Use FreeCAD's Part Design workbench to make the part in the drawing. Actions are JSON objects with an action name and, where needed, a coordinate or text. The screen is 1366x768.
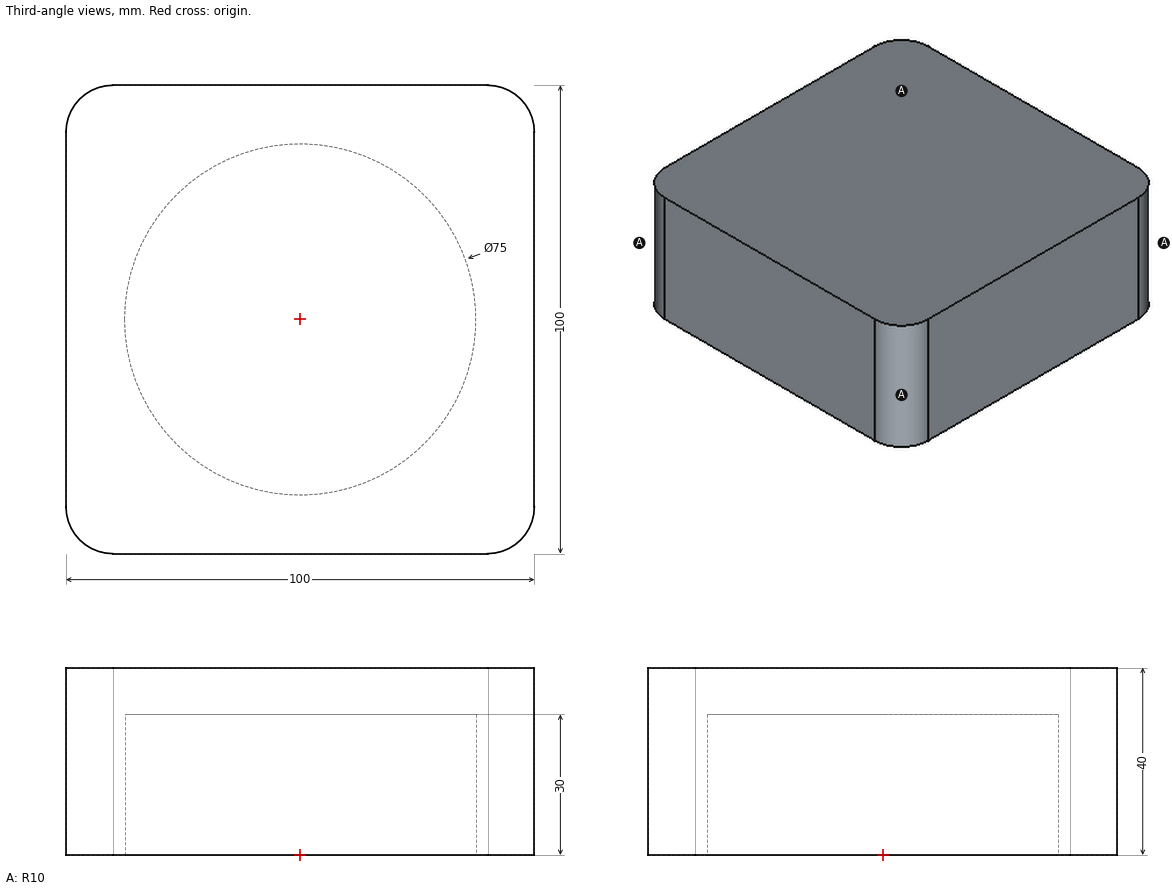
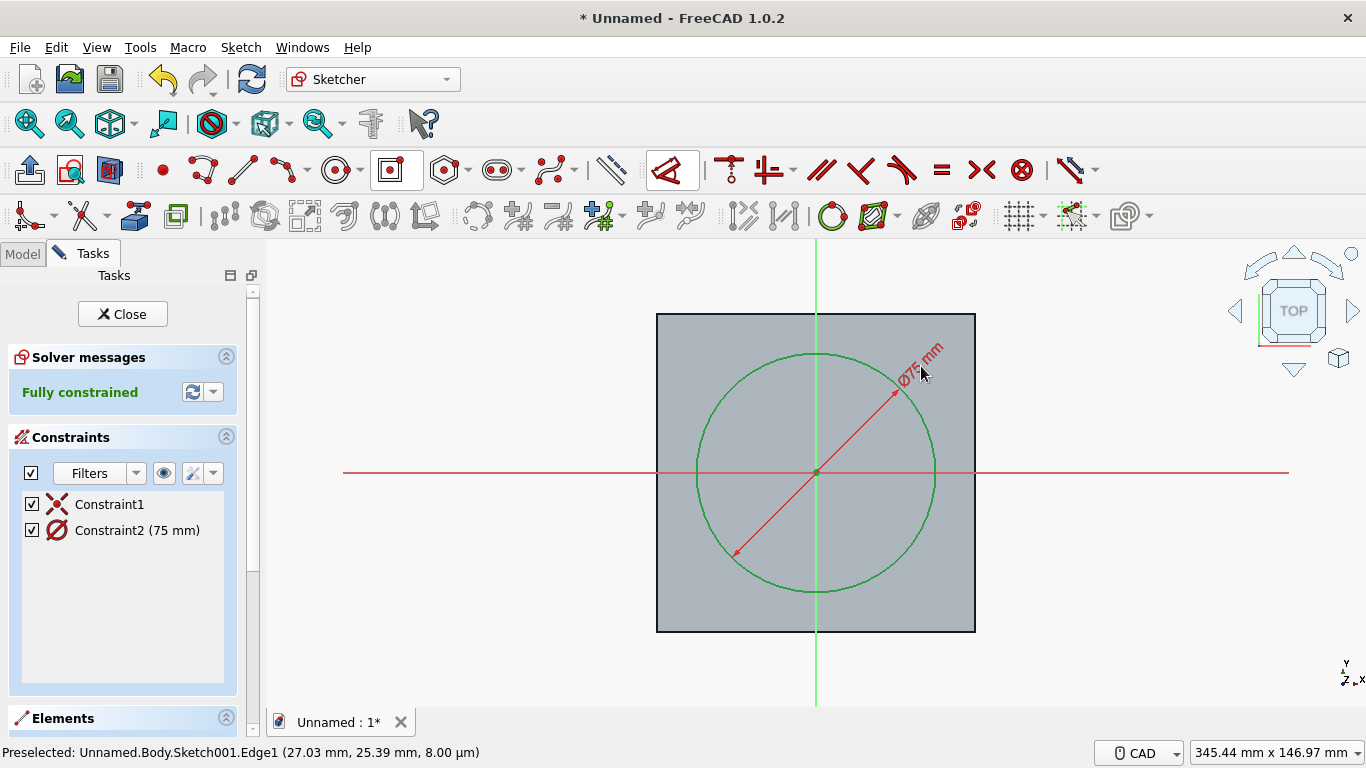
{"action": "left_click", "coordinate": [123, 314]}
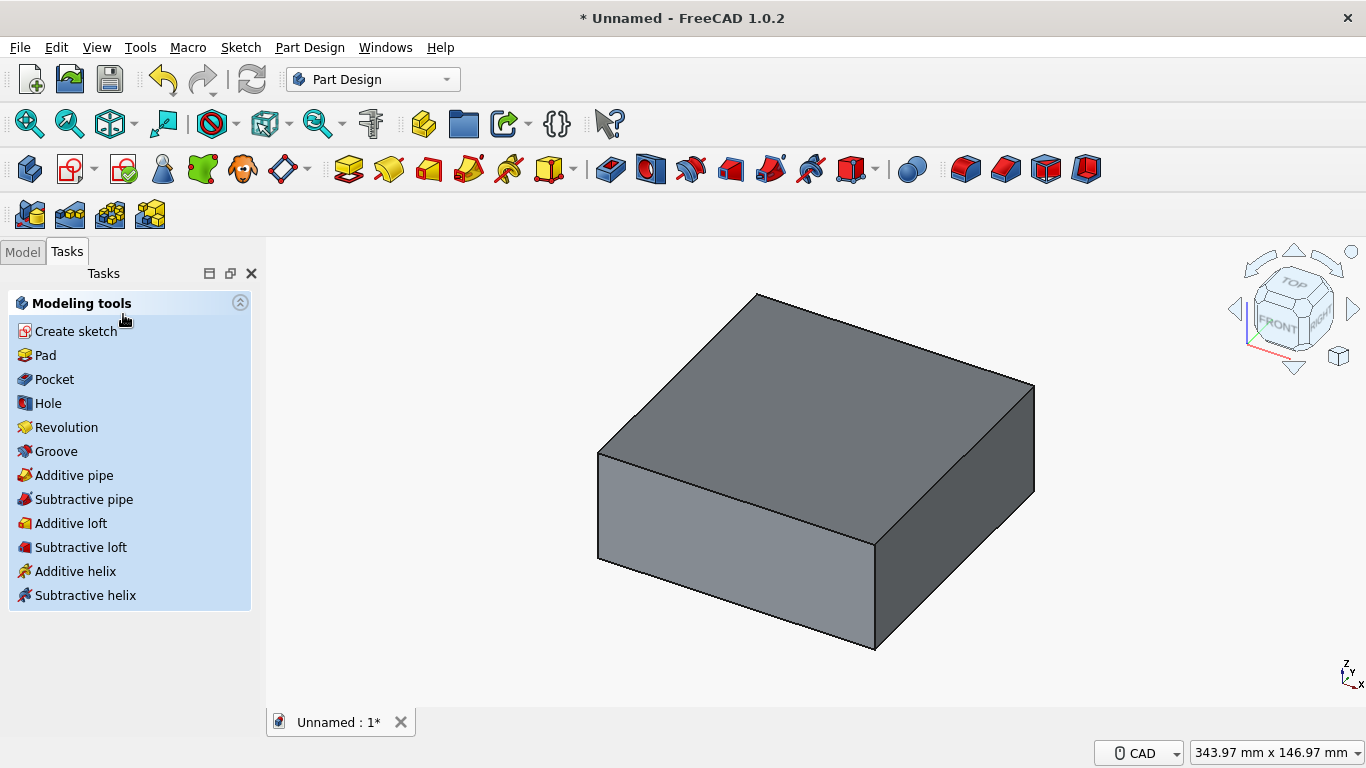
{"action": "left_click", "coordinate": [612, 170]}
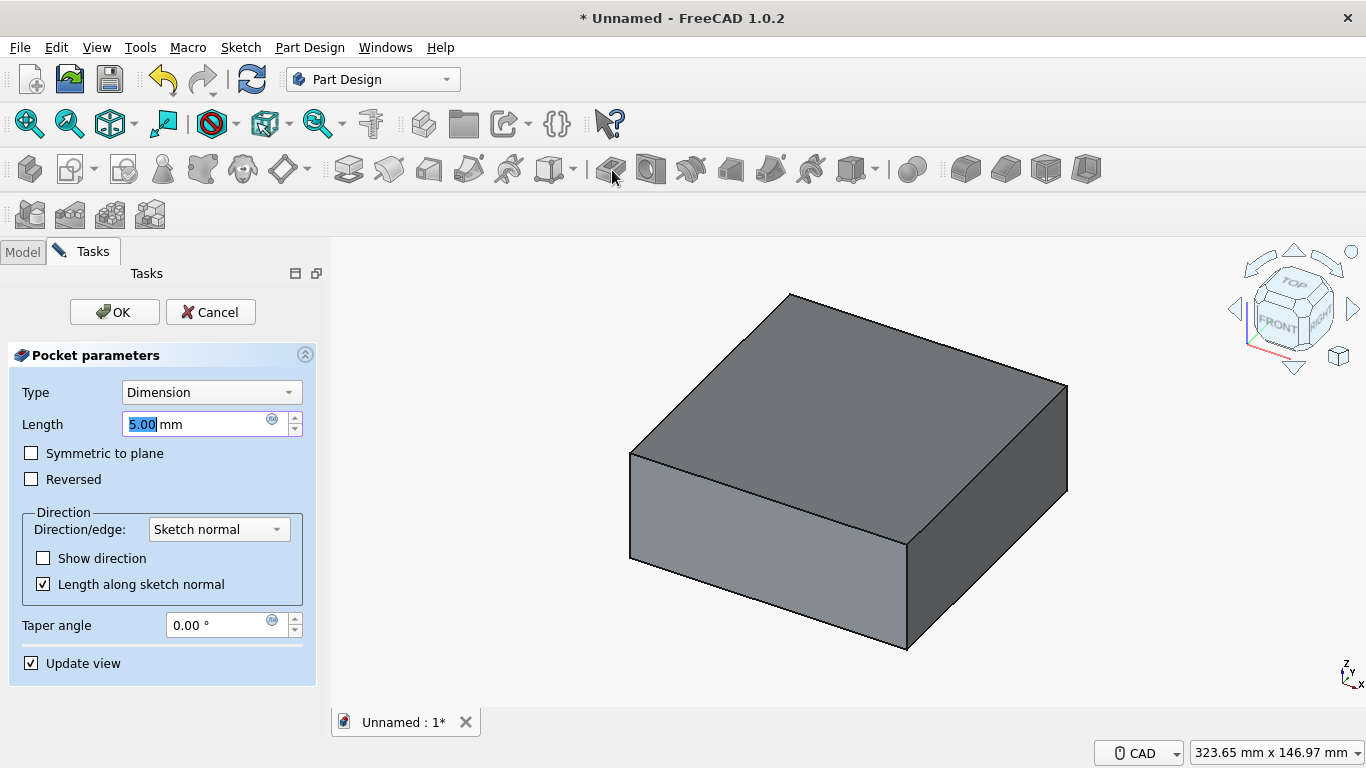
{"action": "type", "text": "30"}
{"action": "key", "text": "Tab"}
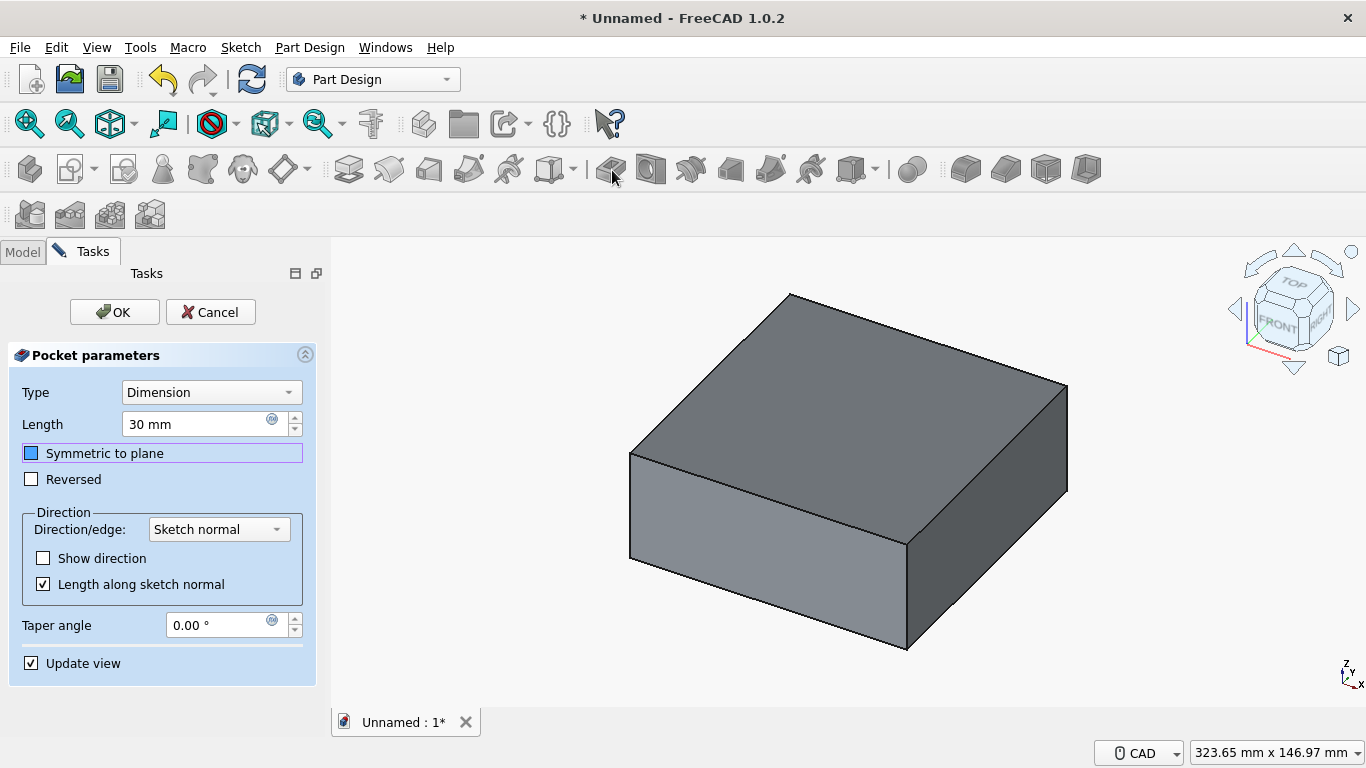
{"action": "left_click", "coordinate": [30, 479]}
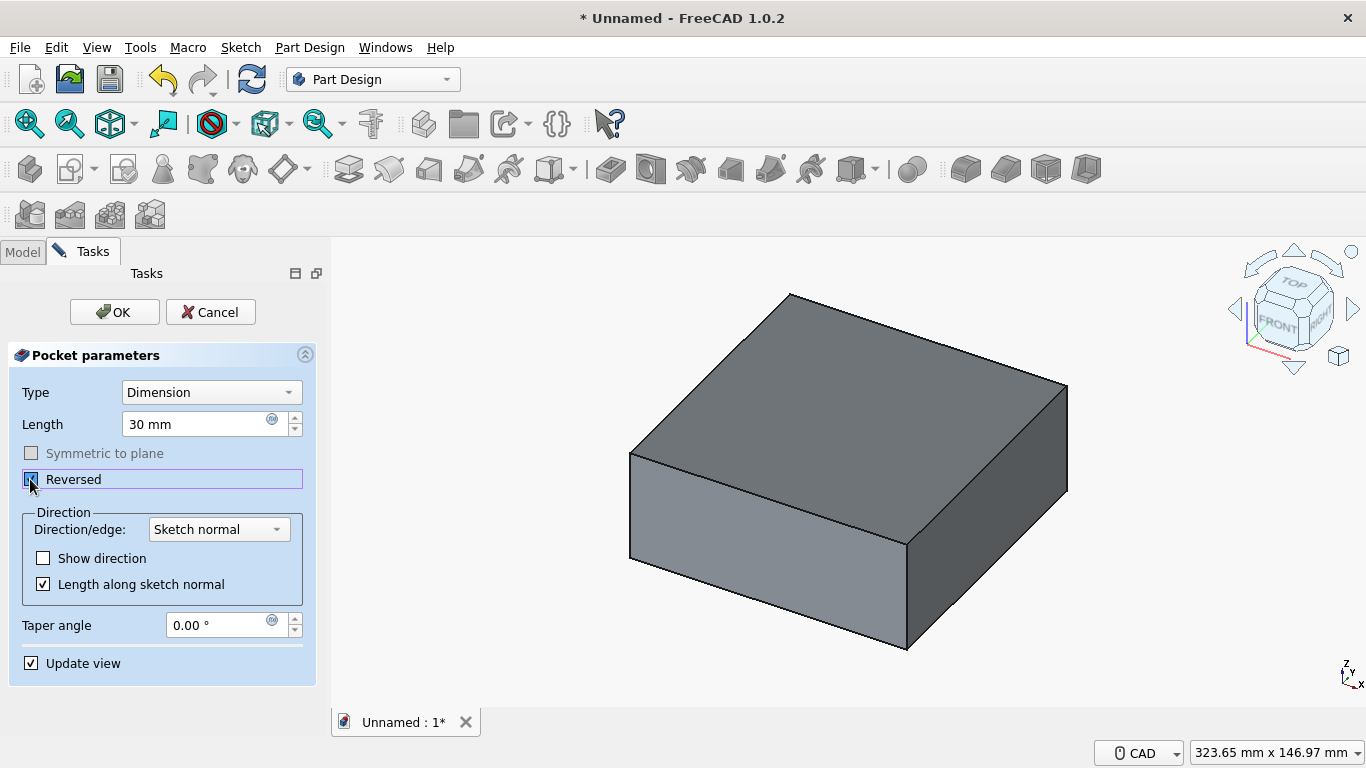
{"action": "left_click", "coordinate": [115, 312]}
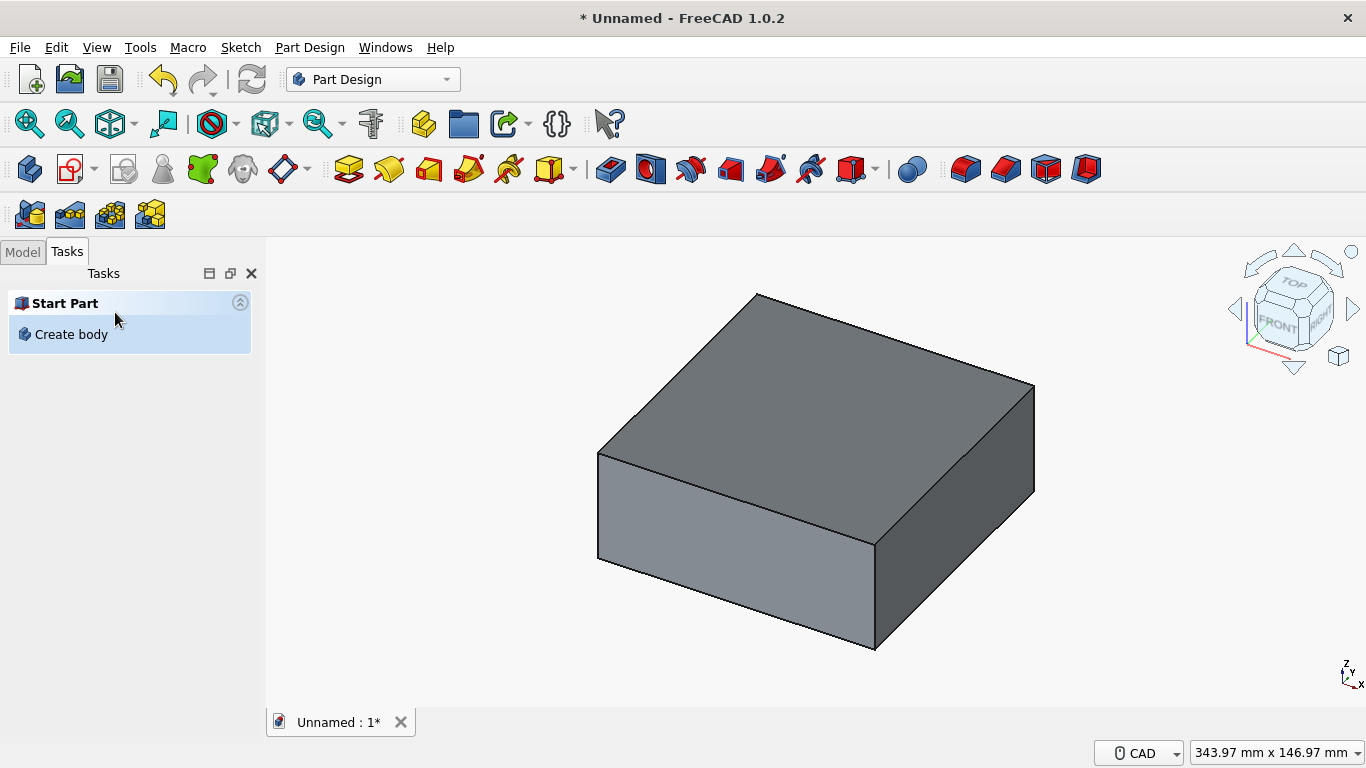
{"action": "left_click", "coordinate": [875, 596]}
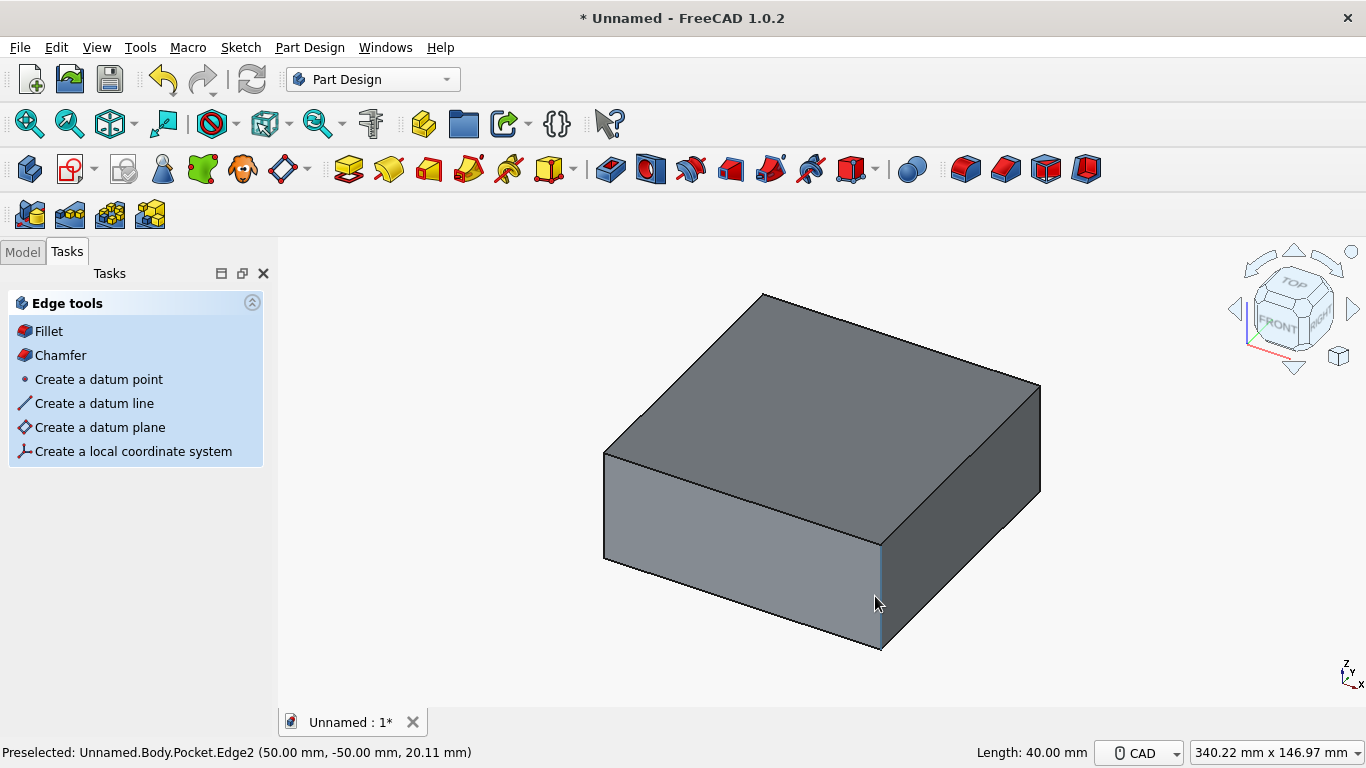
{"action": "key", "text": "0"}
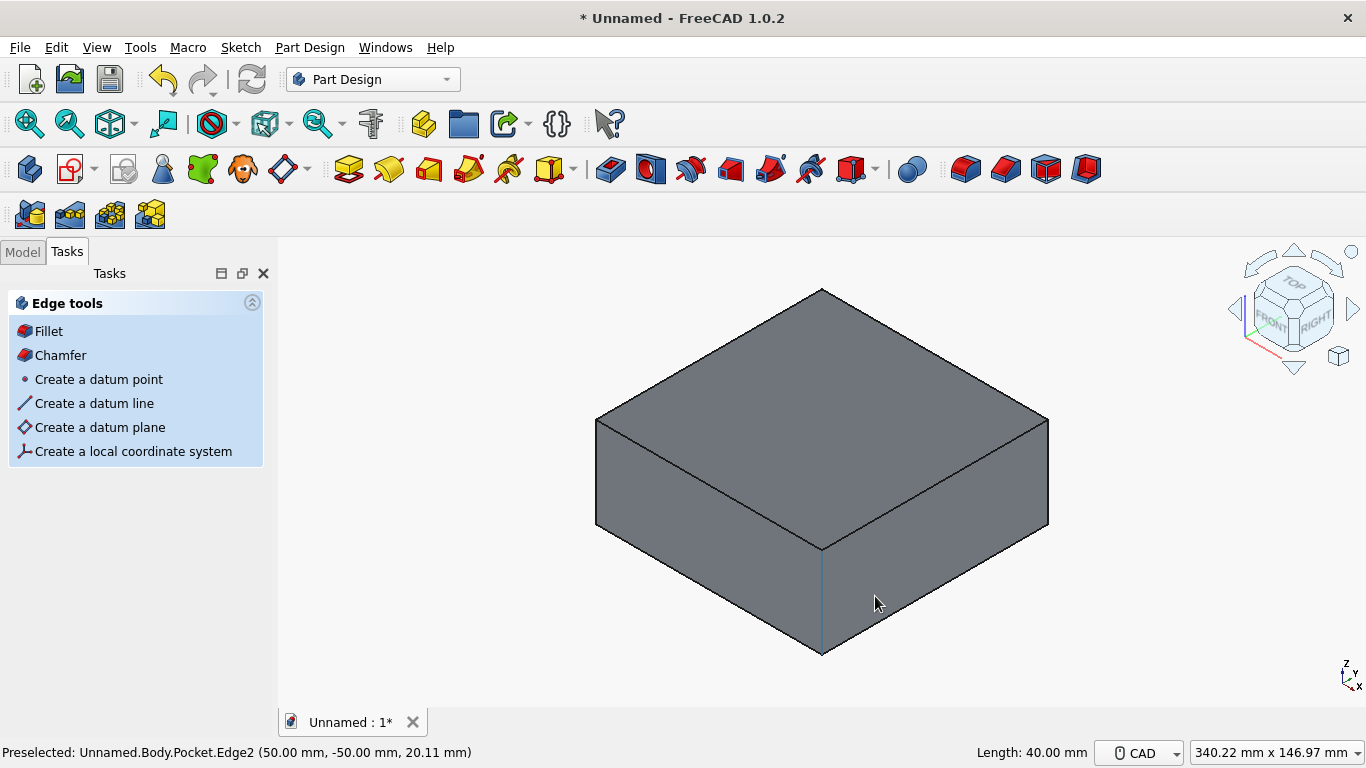
{"action": "key", "text": "2"}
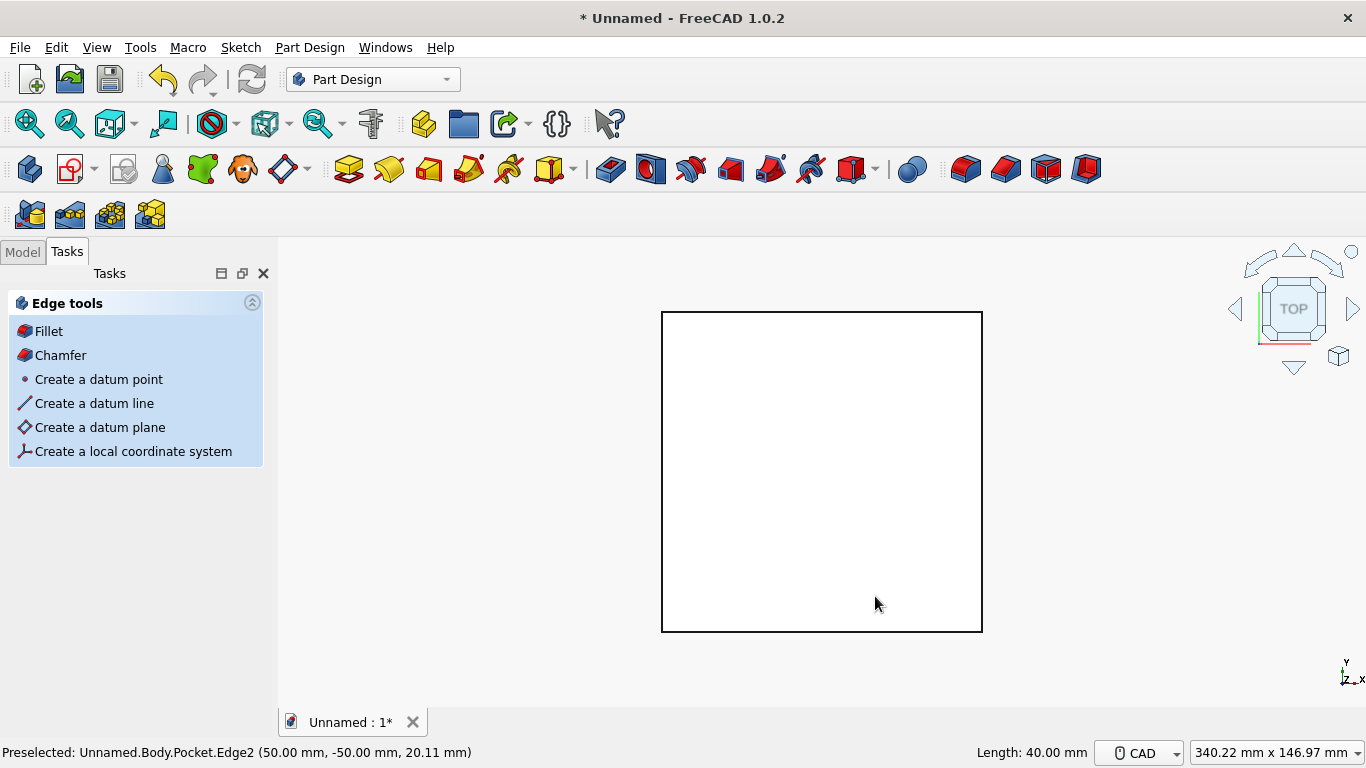
{"action": "key", "text": "1"}